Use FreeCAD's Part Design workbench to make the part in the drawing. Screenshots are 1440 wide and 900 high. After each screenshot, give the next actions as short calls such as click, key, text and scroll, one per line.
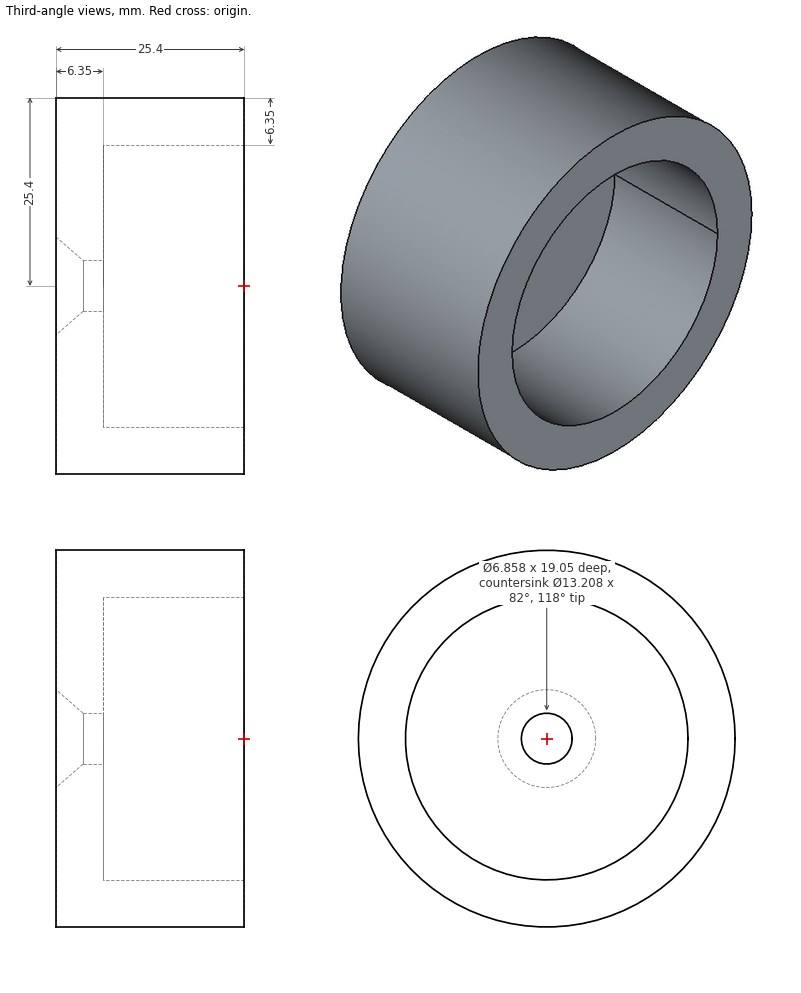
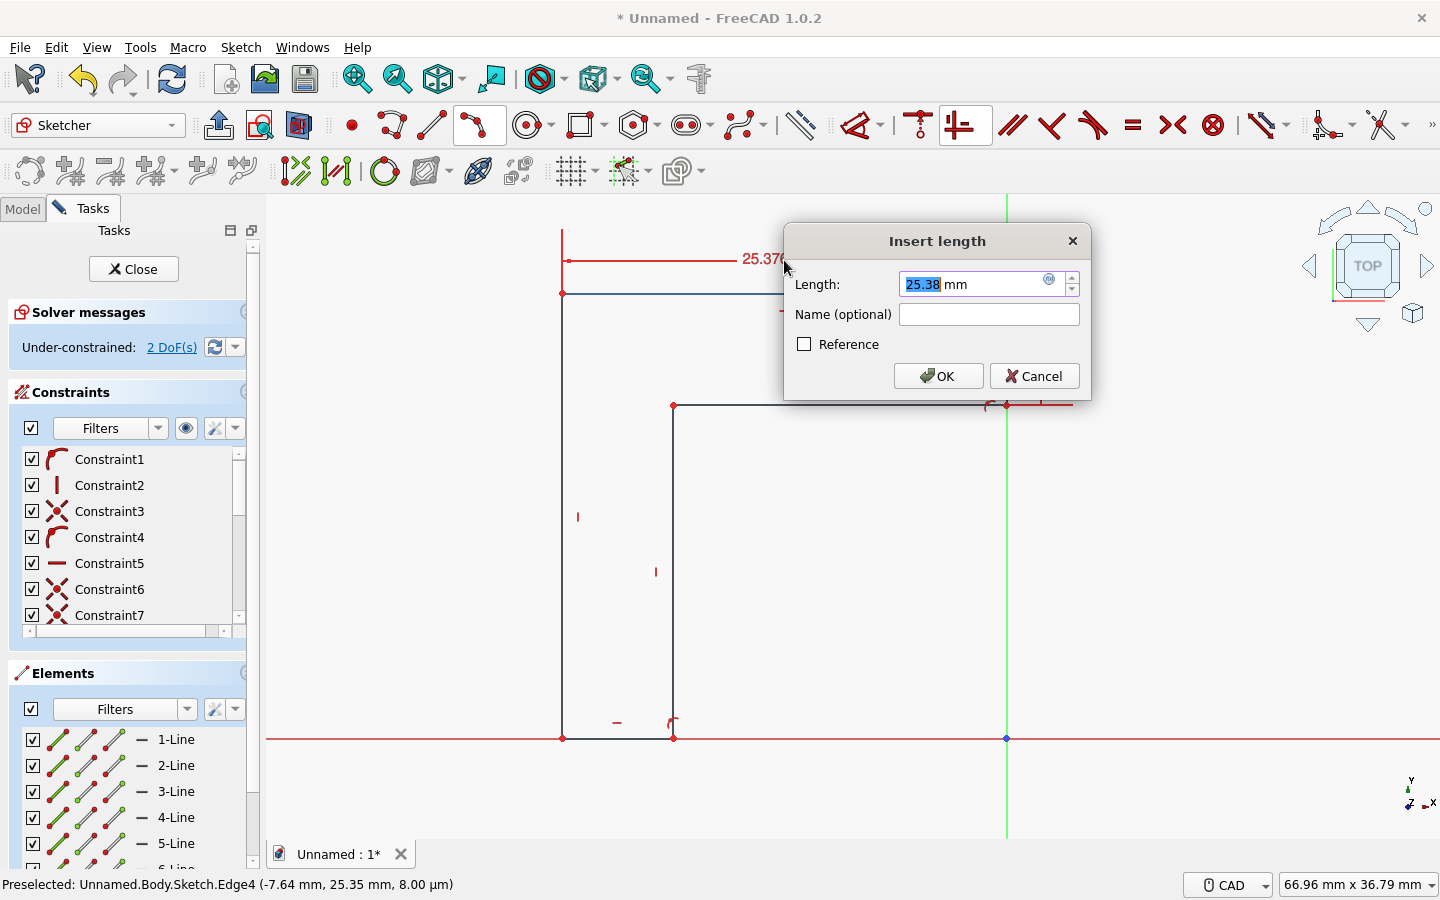
text(25.4)
key(Return)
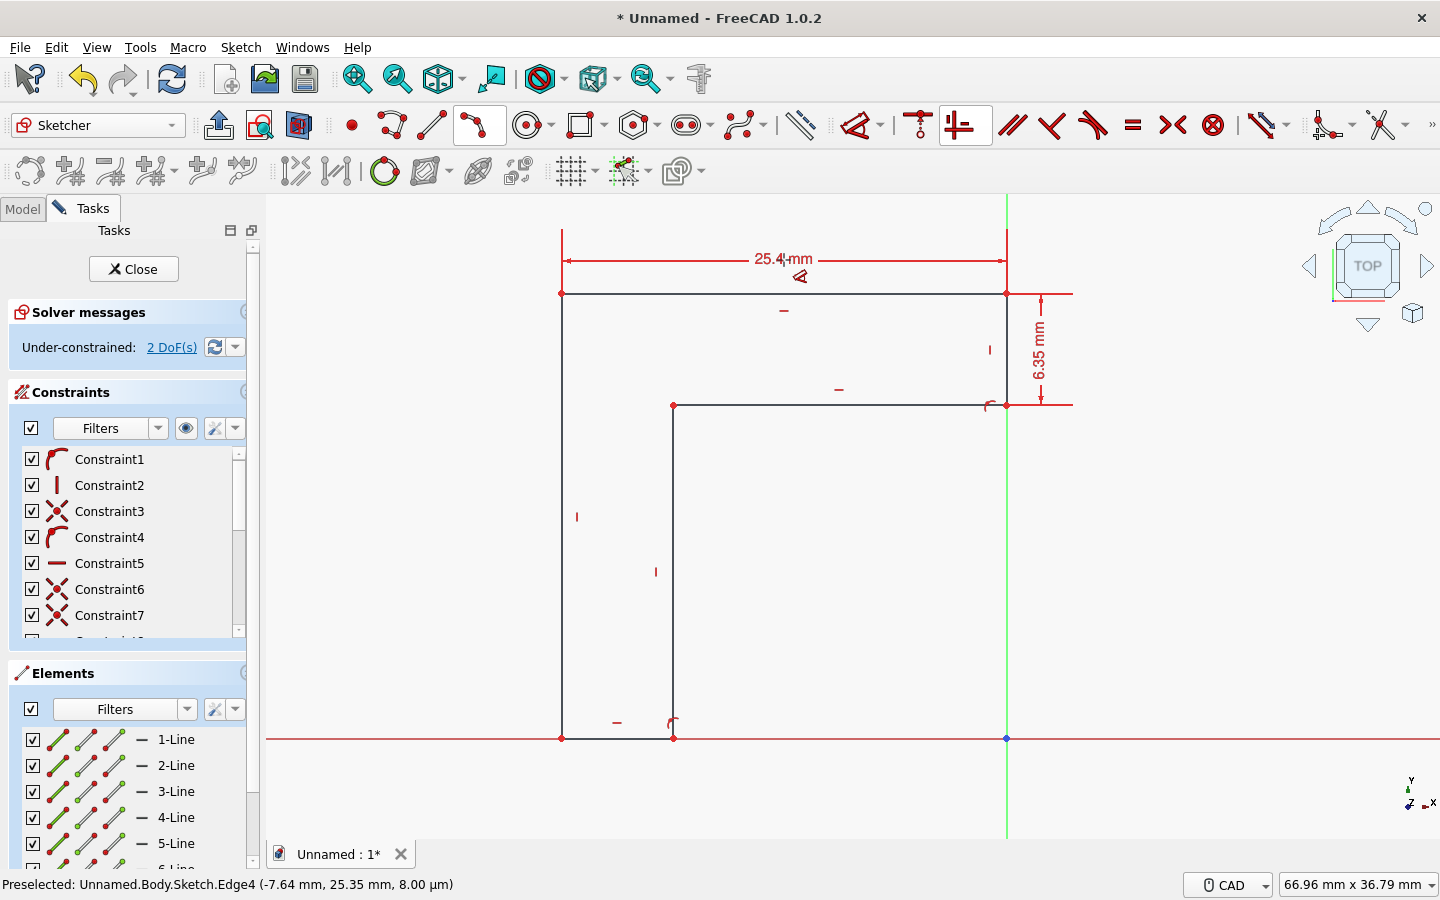
click(562, 427)
click(528, 516)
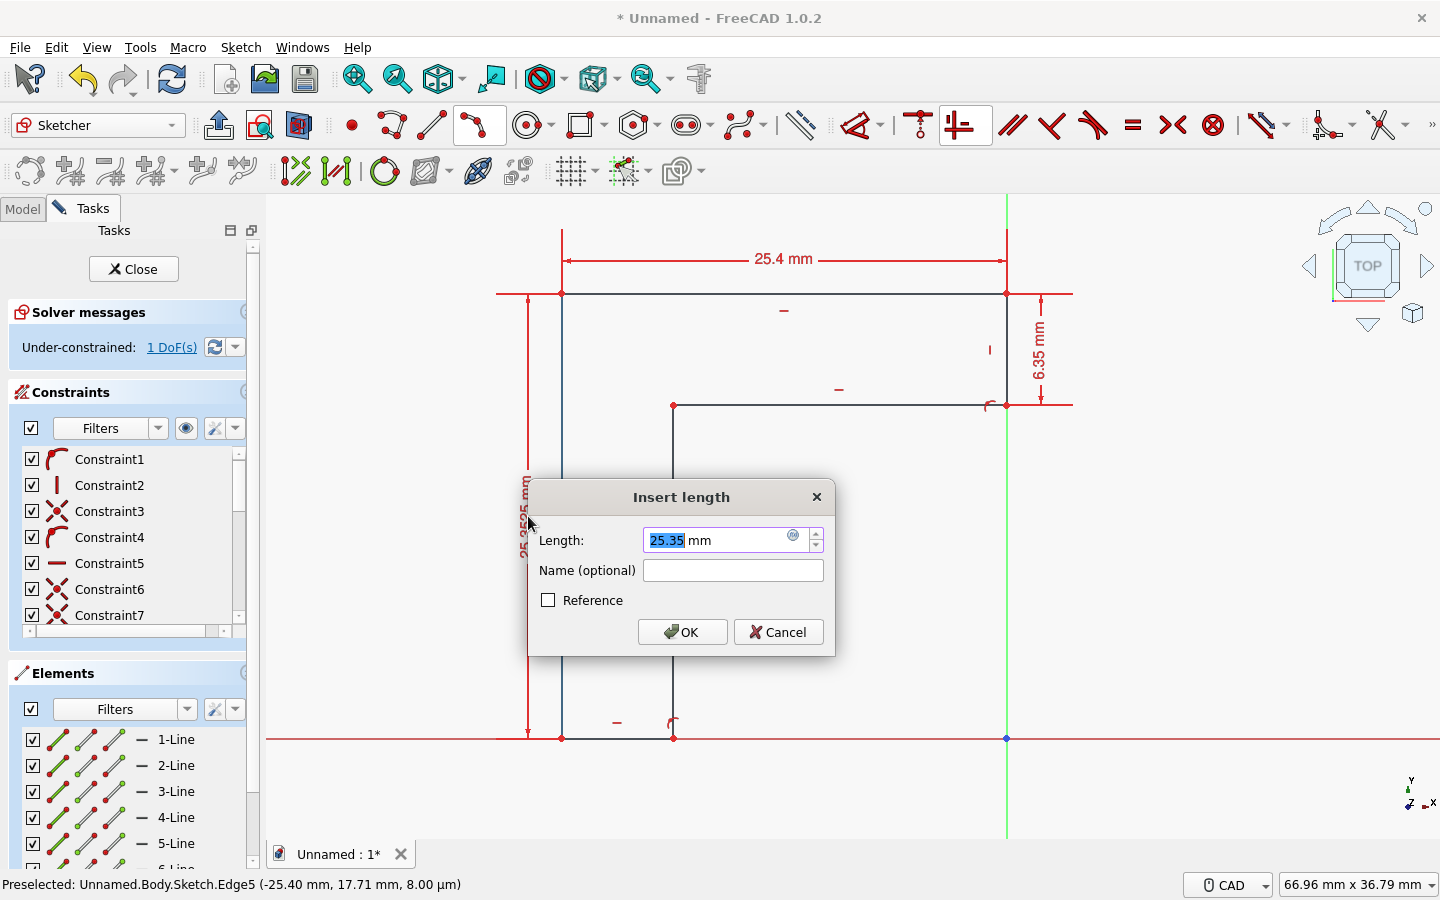
text(25.4)
key(Return)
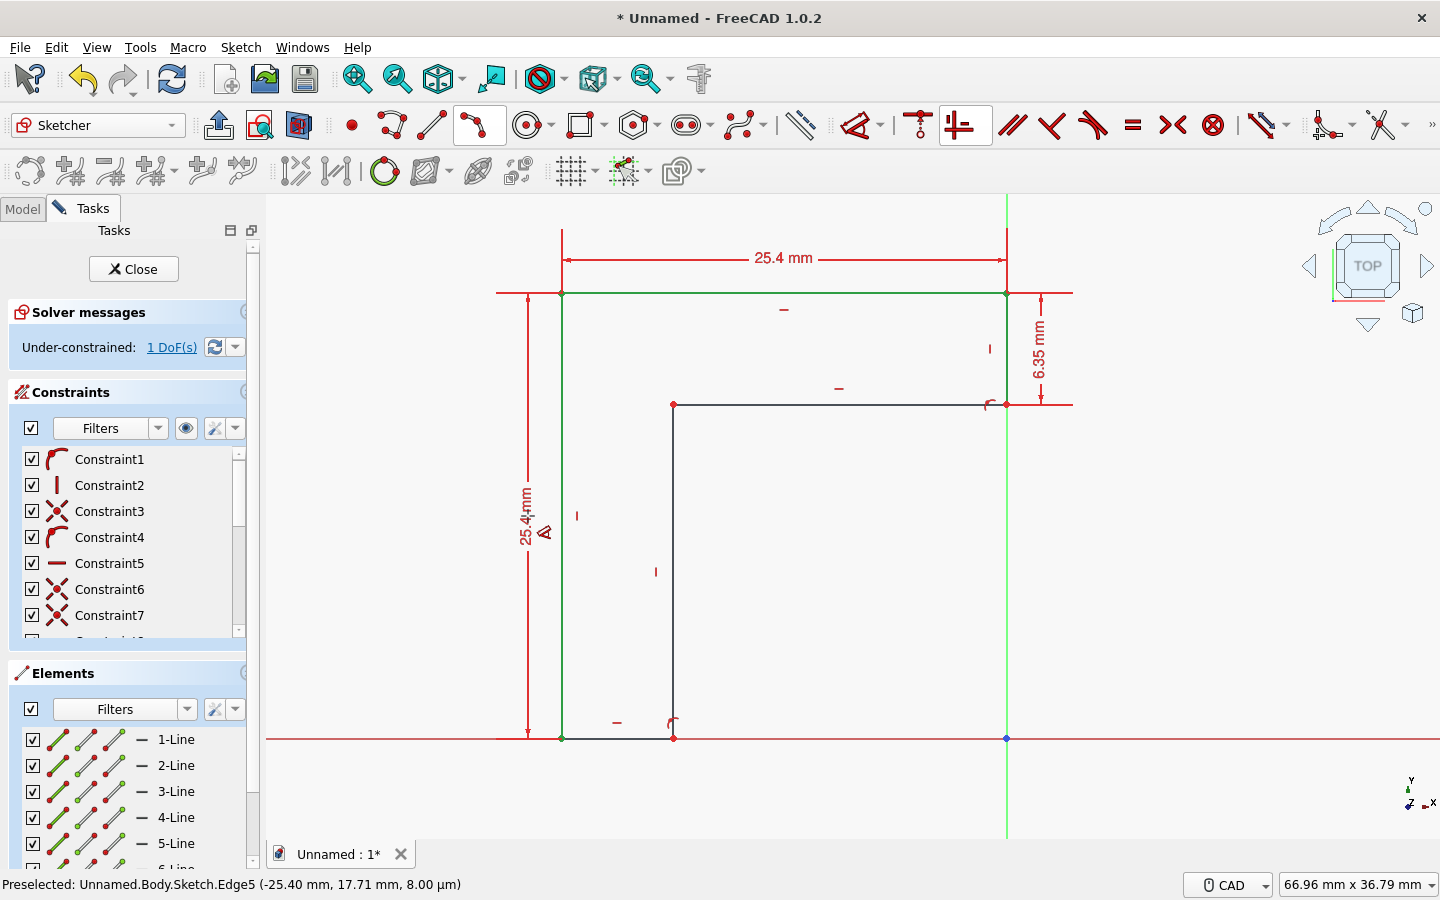
click(595, 739)
click(617, 773)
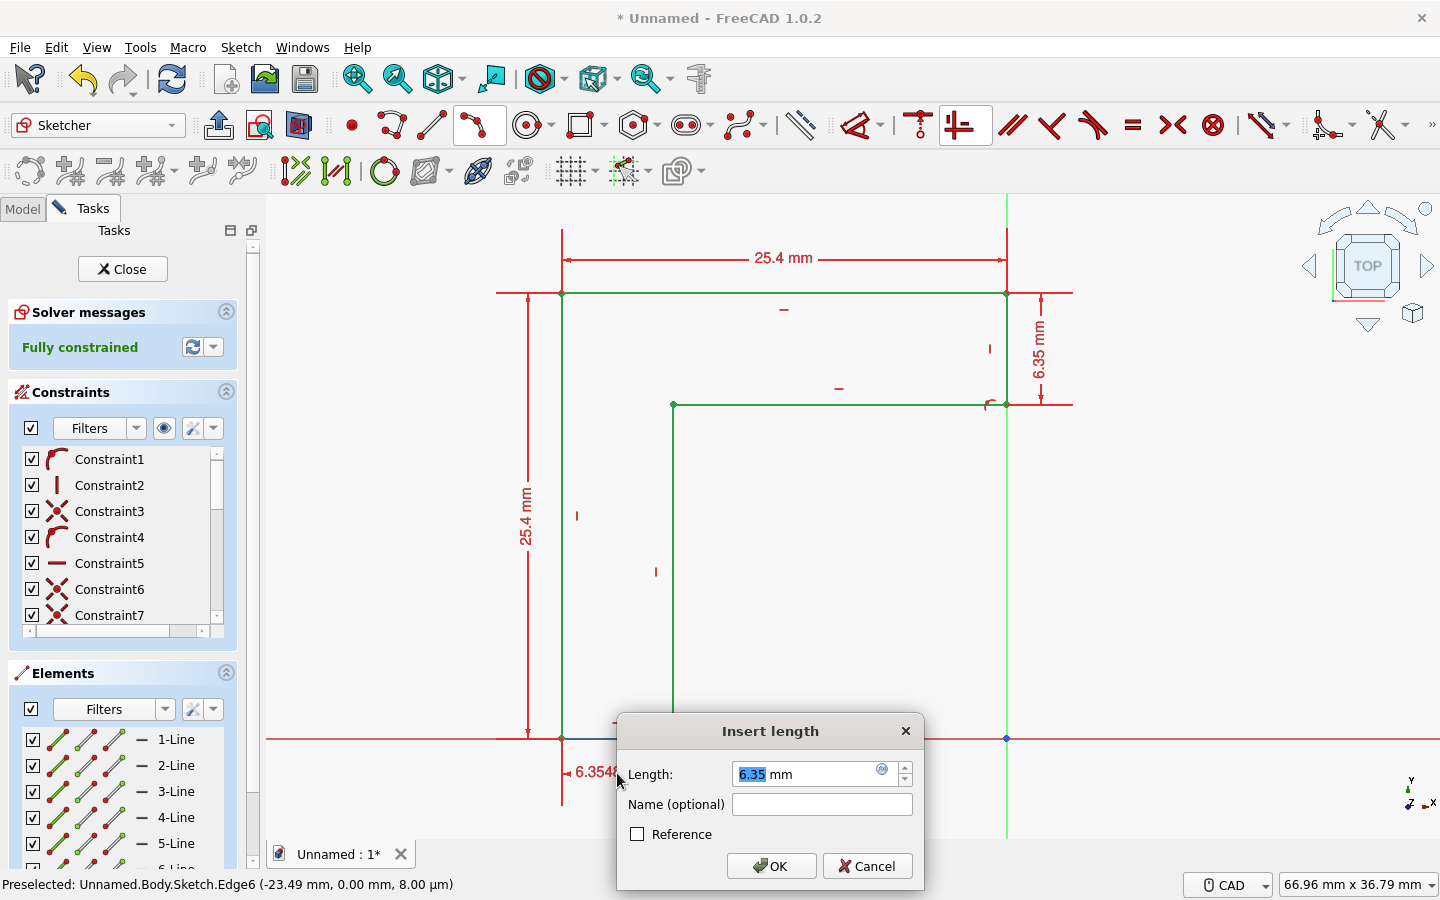
text(6.35)
key(Return)
key(Escape)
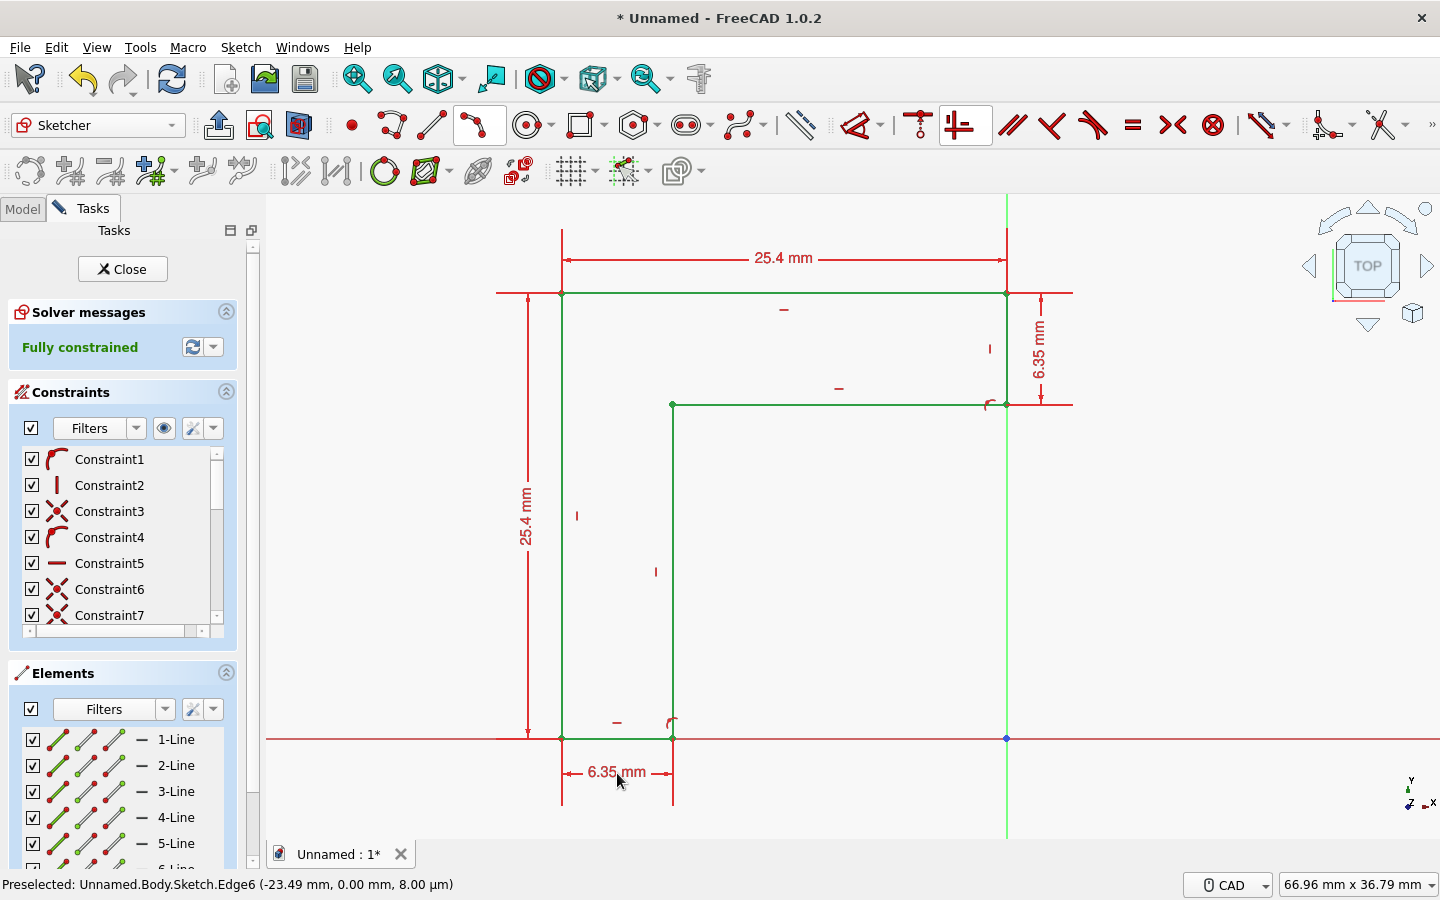
click(123, 269)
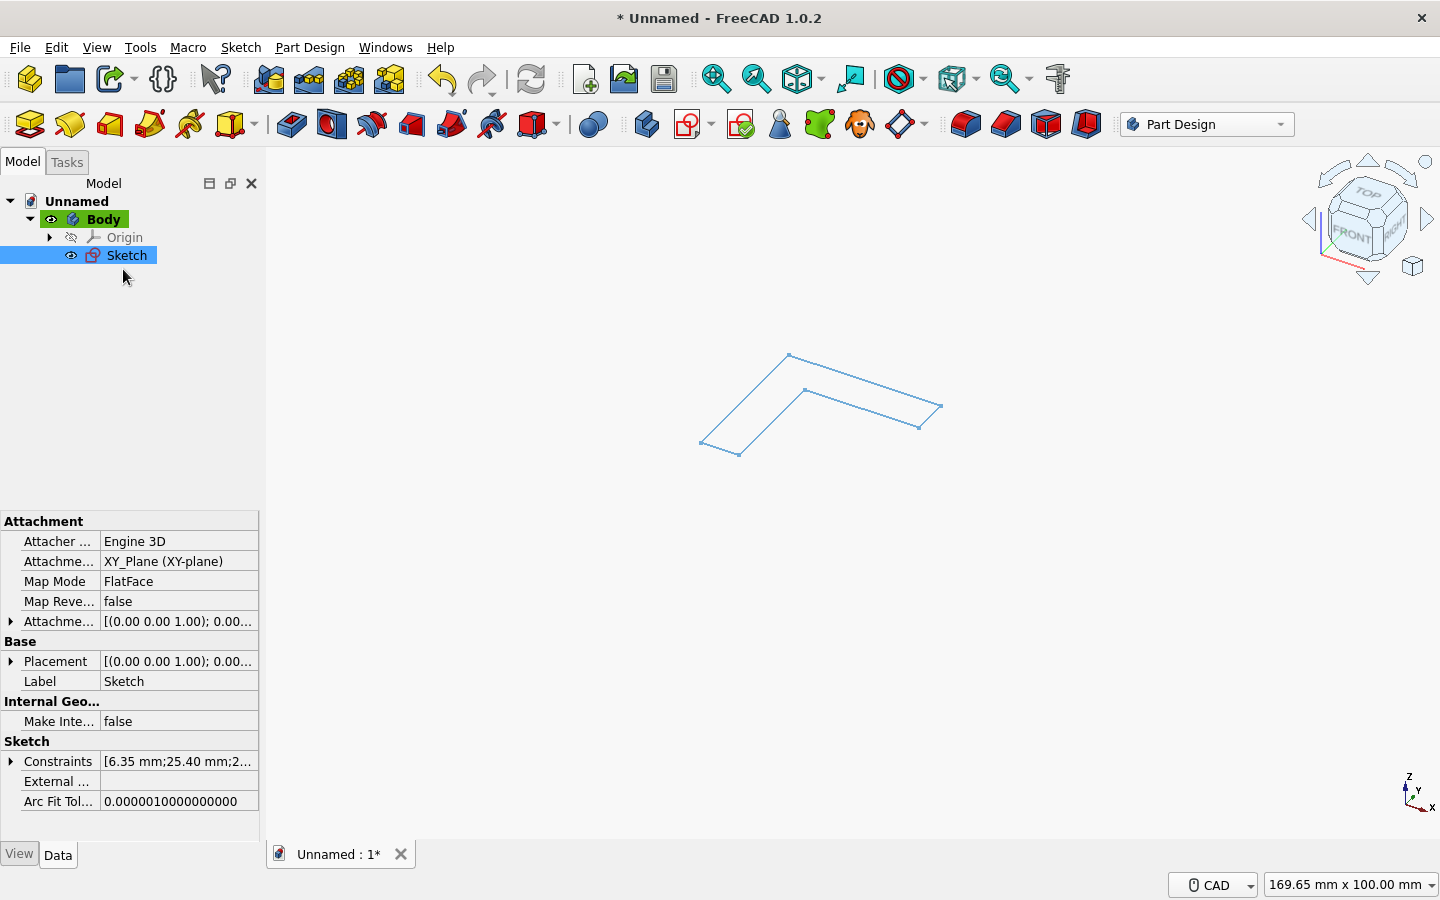
click(70, 124)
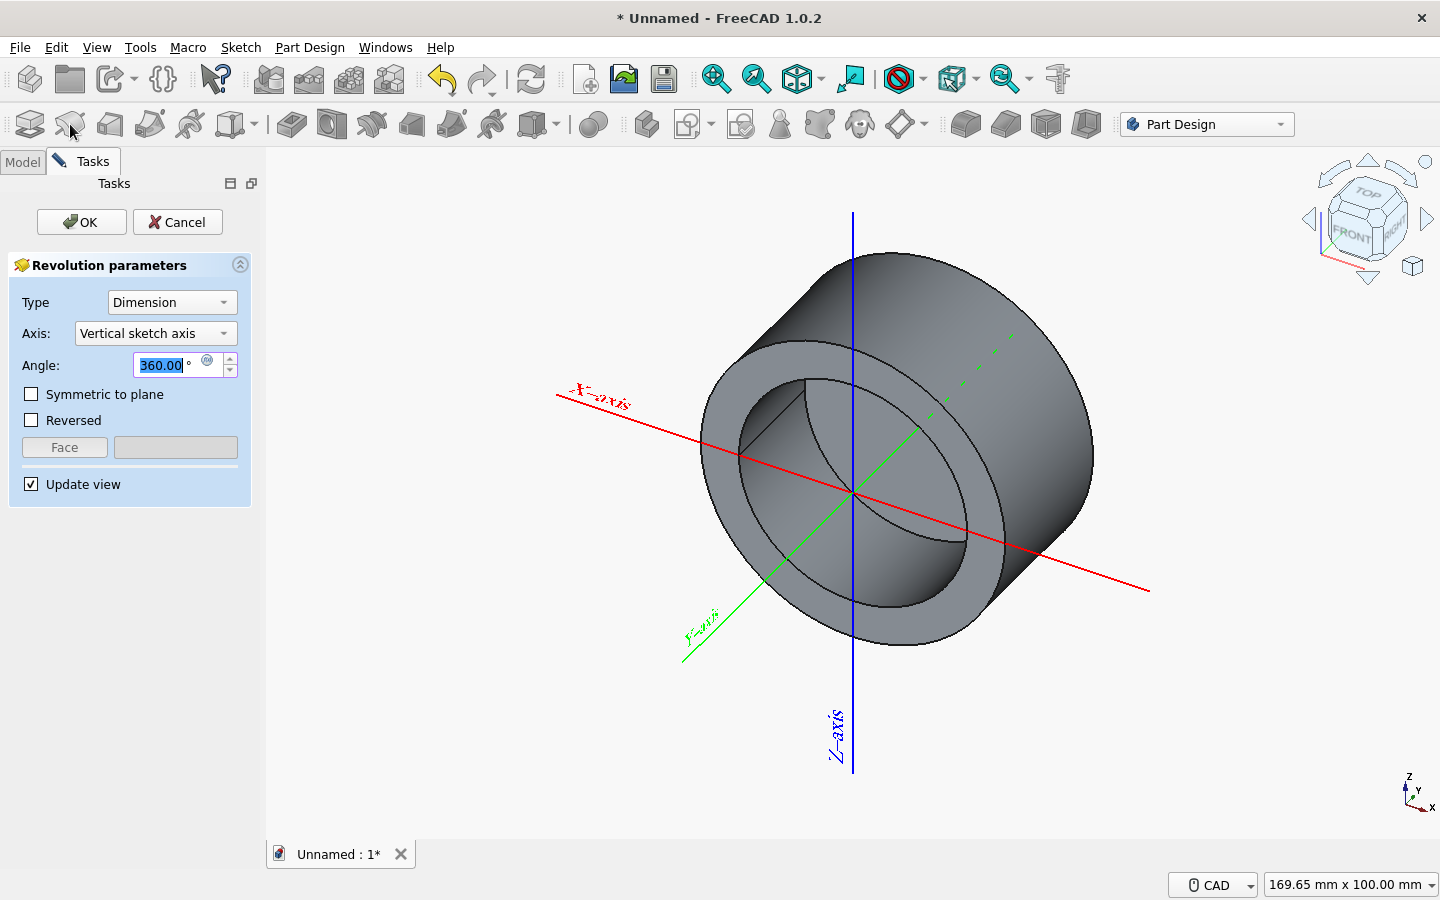
click(156, 334)